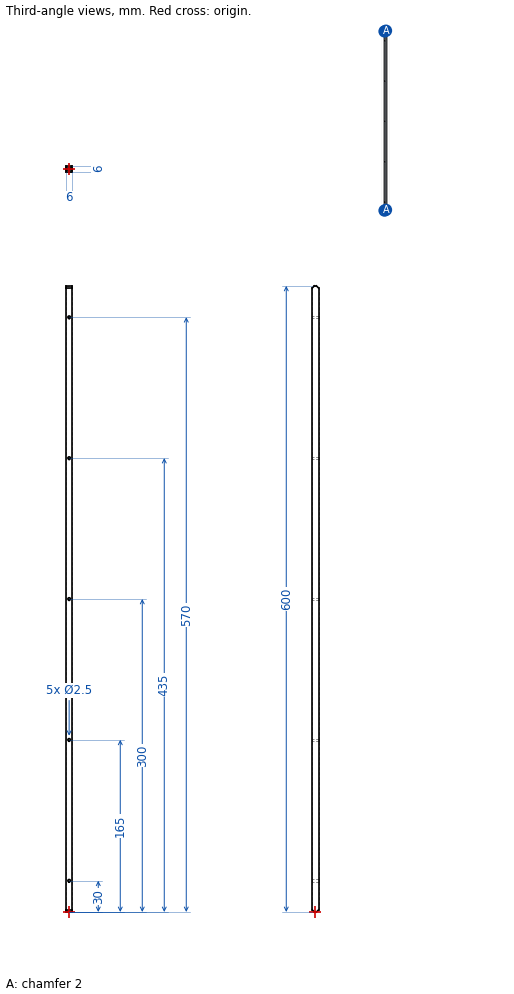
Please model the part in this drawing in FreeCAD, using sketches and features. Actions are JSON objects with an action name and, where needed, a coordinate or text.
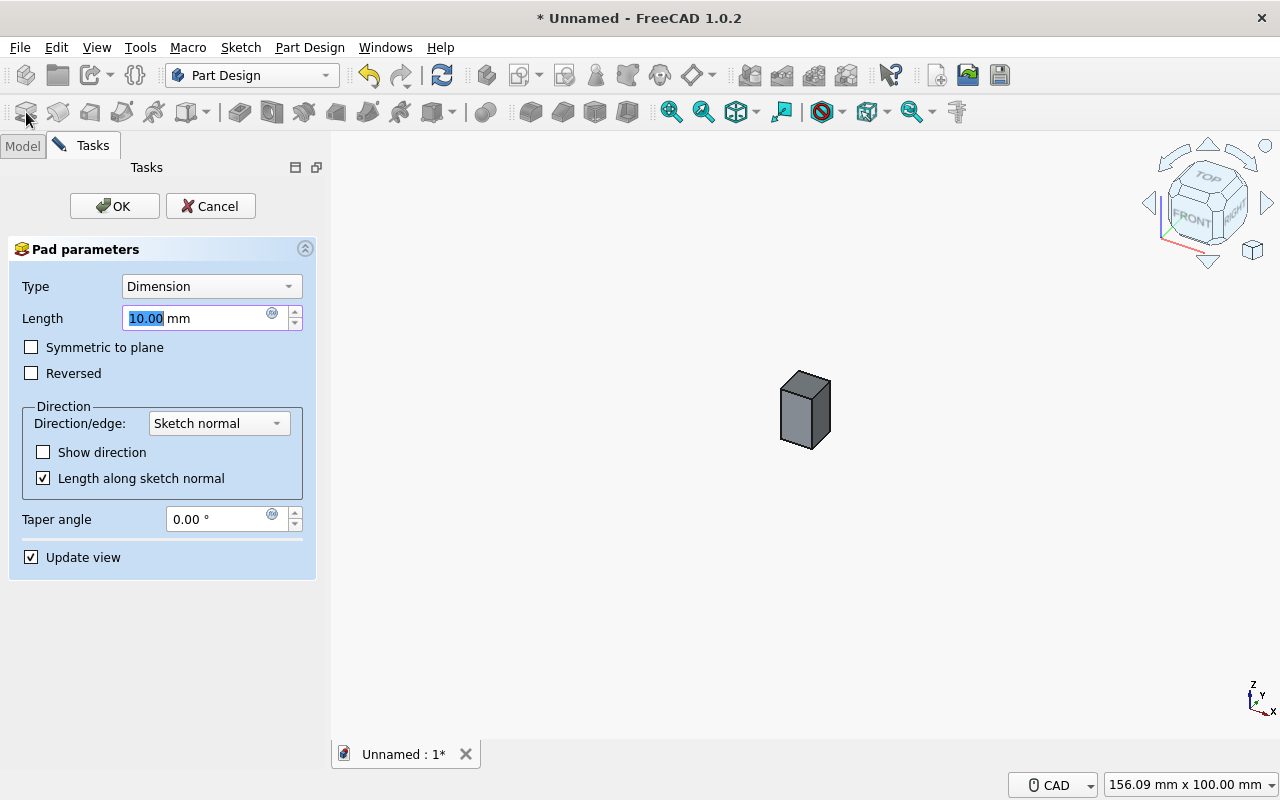
{"action": "type", "text": "600"}
{"action": "key", "text": "Tab"}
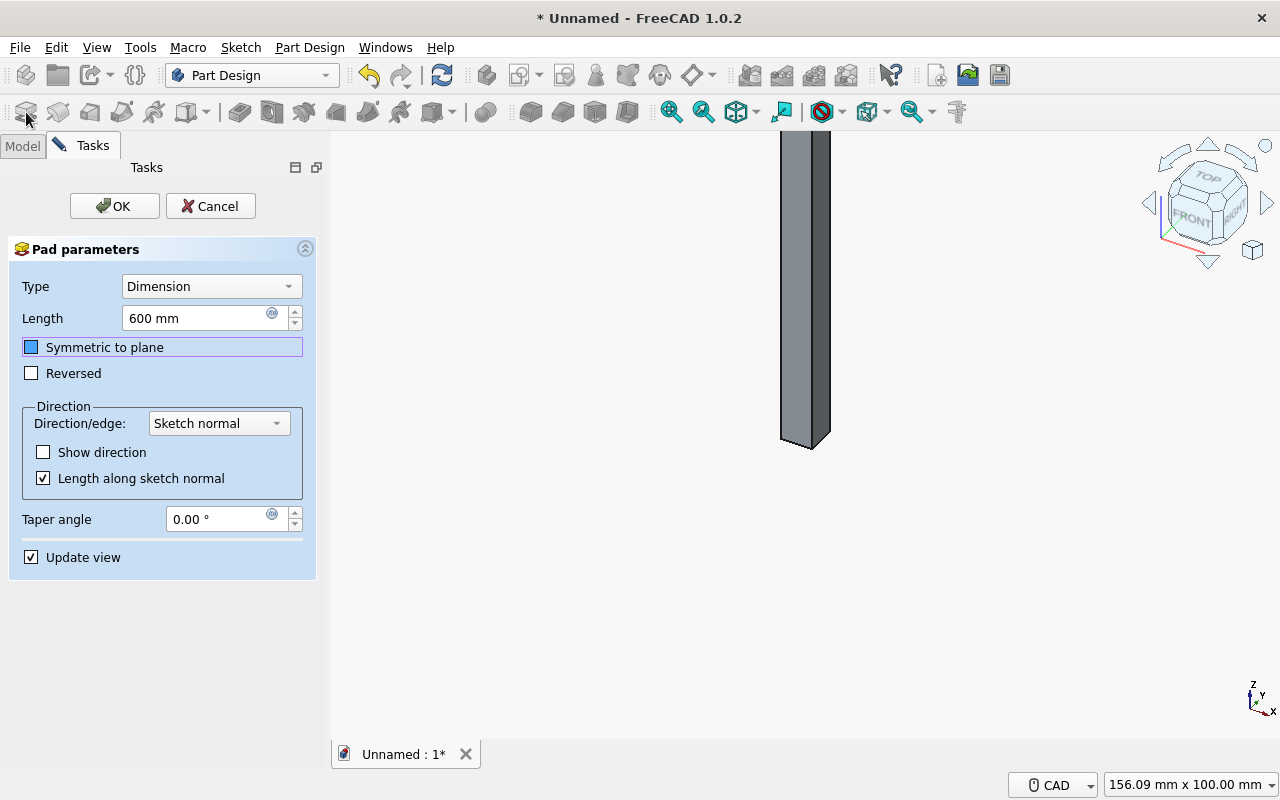
{"action": "left_click", "coordinate": [115, 206]}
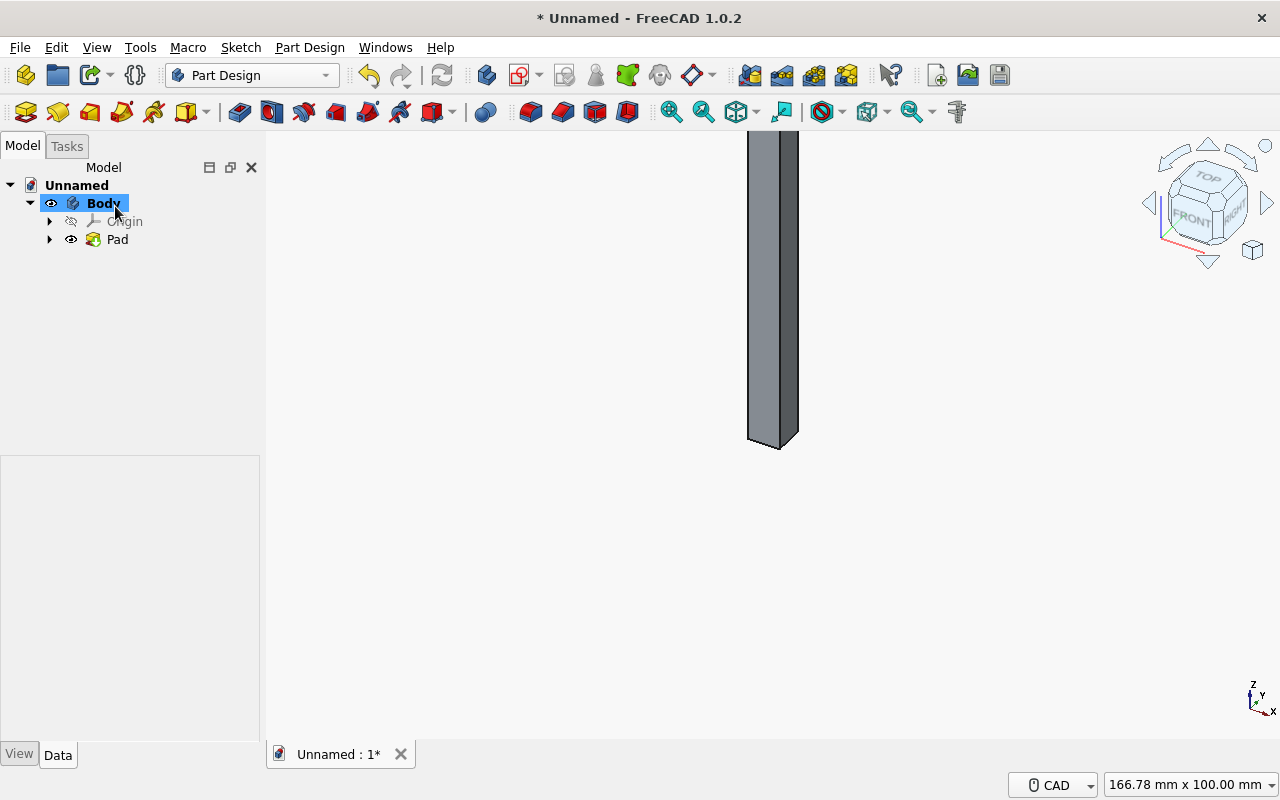
{"action": "left_click", "coordinate": [672, 112]}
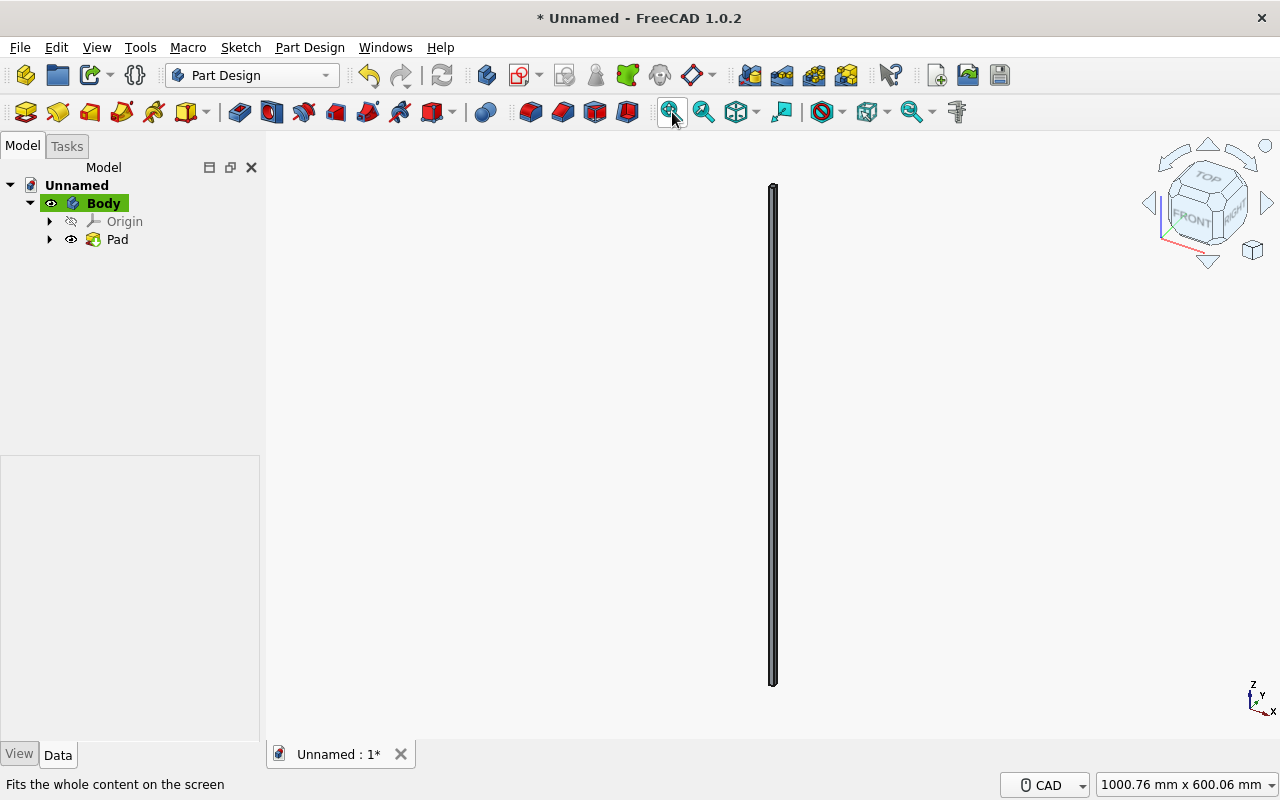
{"action": "key", "text": "4"}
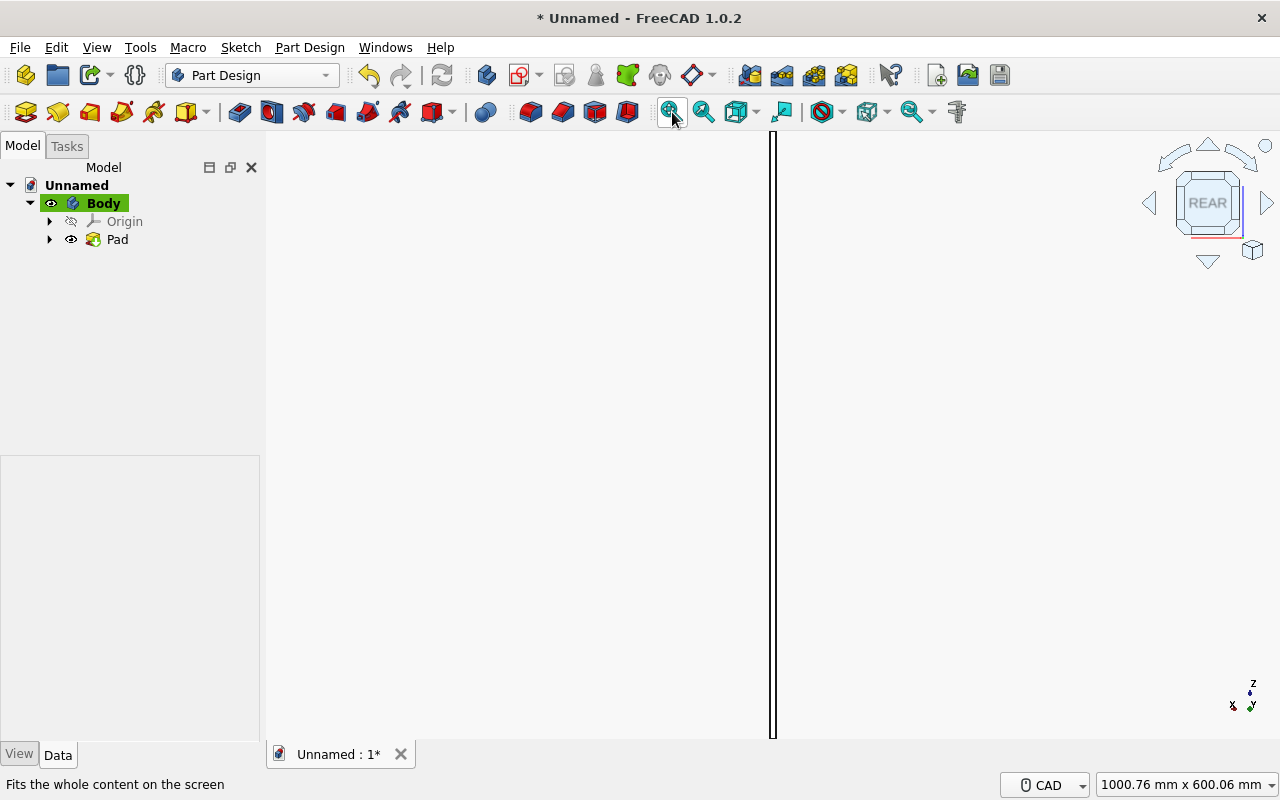
{"action": "left_click", "coordinate": [672, 112]}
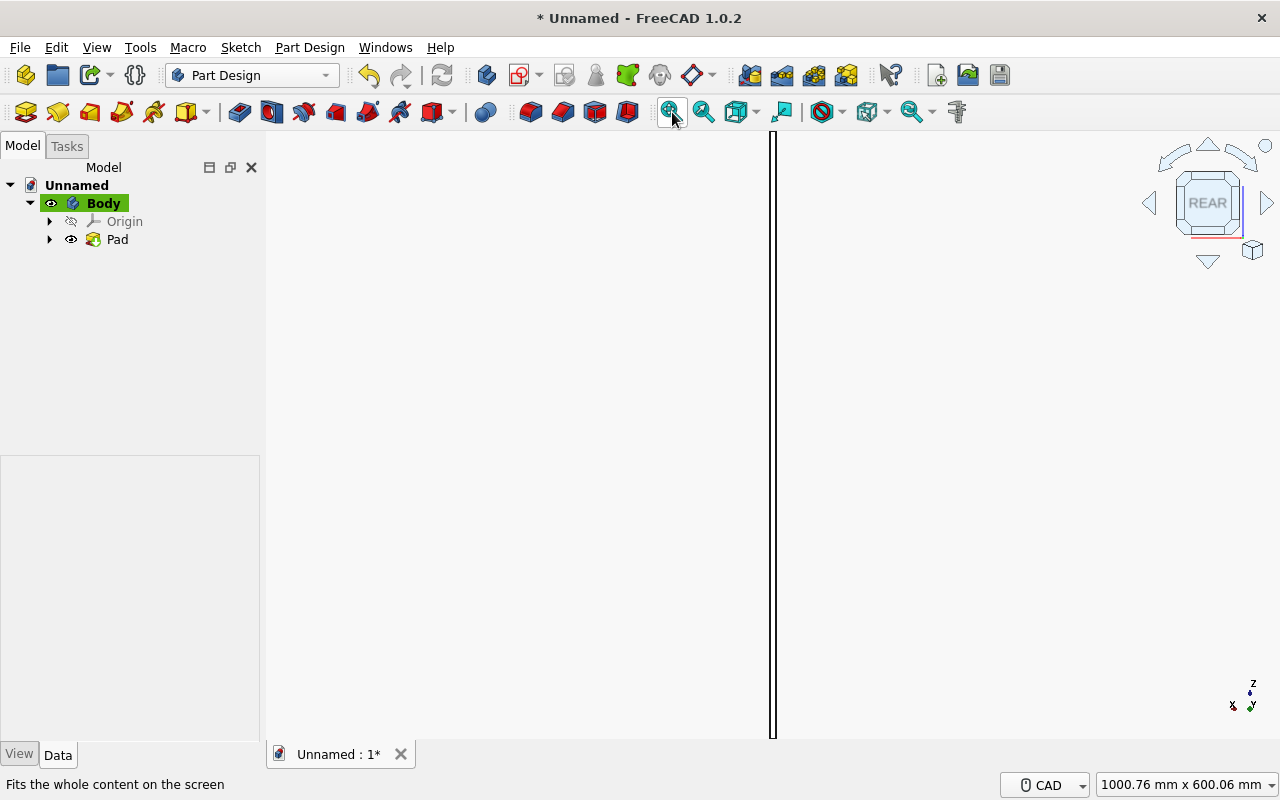
{"action": "scroll", "coordinate": [773, 173], "scroll_direction": "up", "scroll_amount": 7}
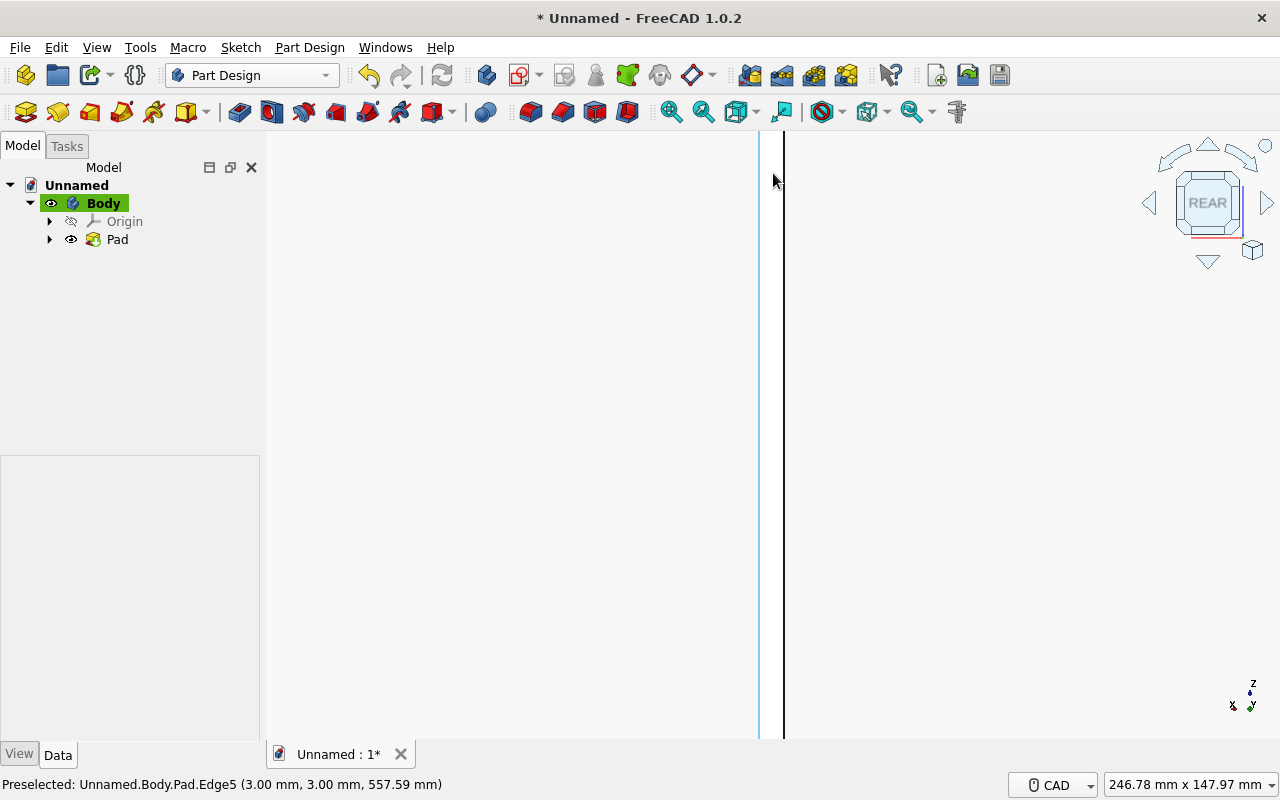
{"action": "left_click", "coordinate": [771, 178]}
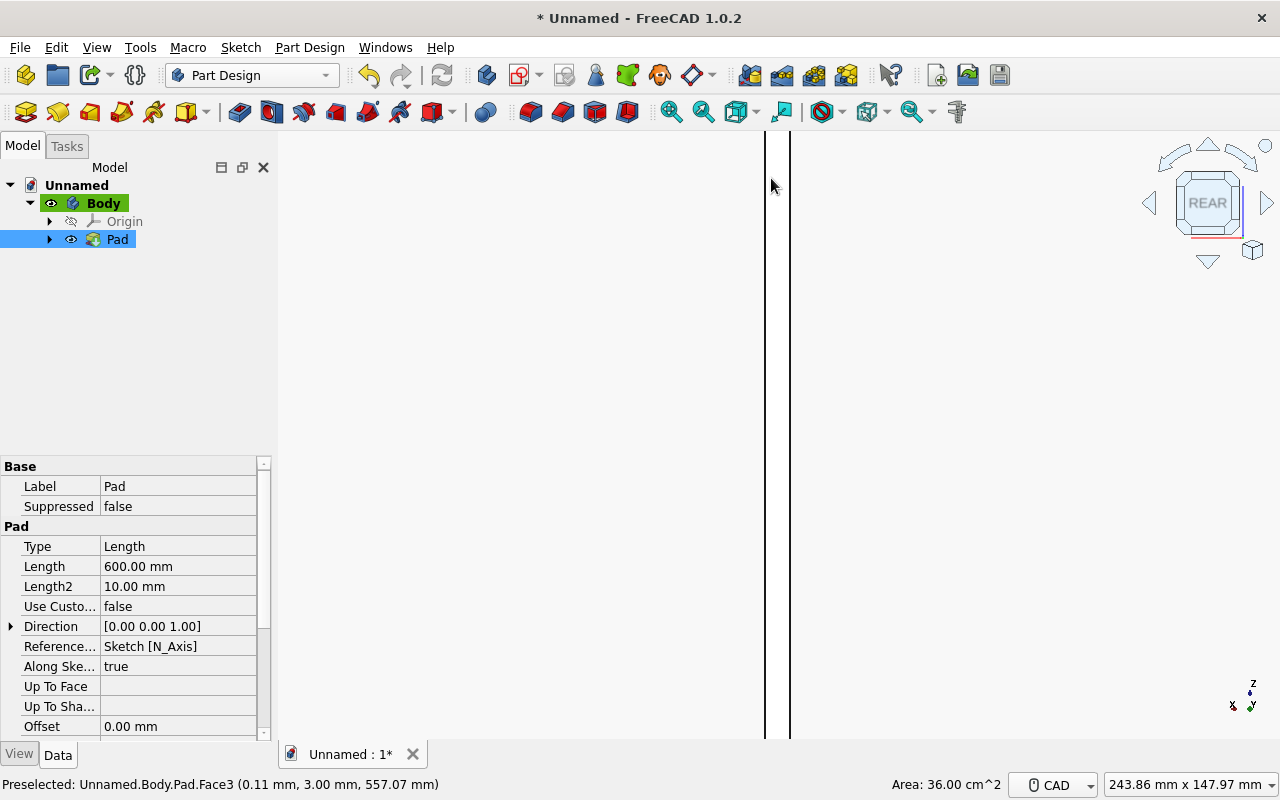
{"action": "left_click", "coordinate": [520, 76]}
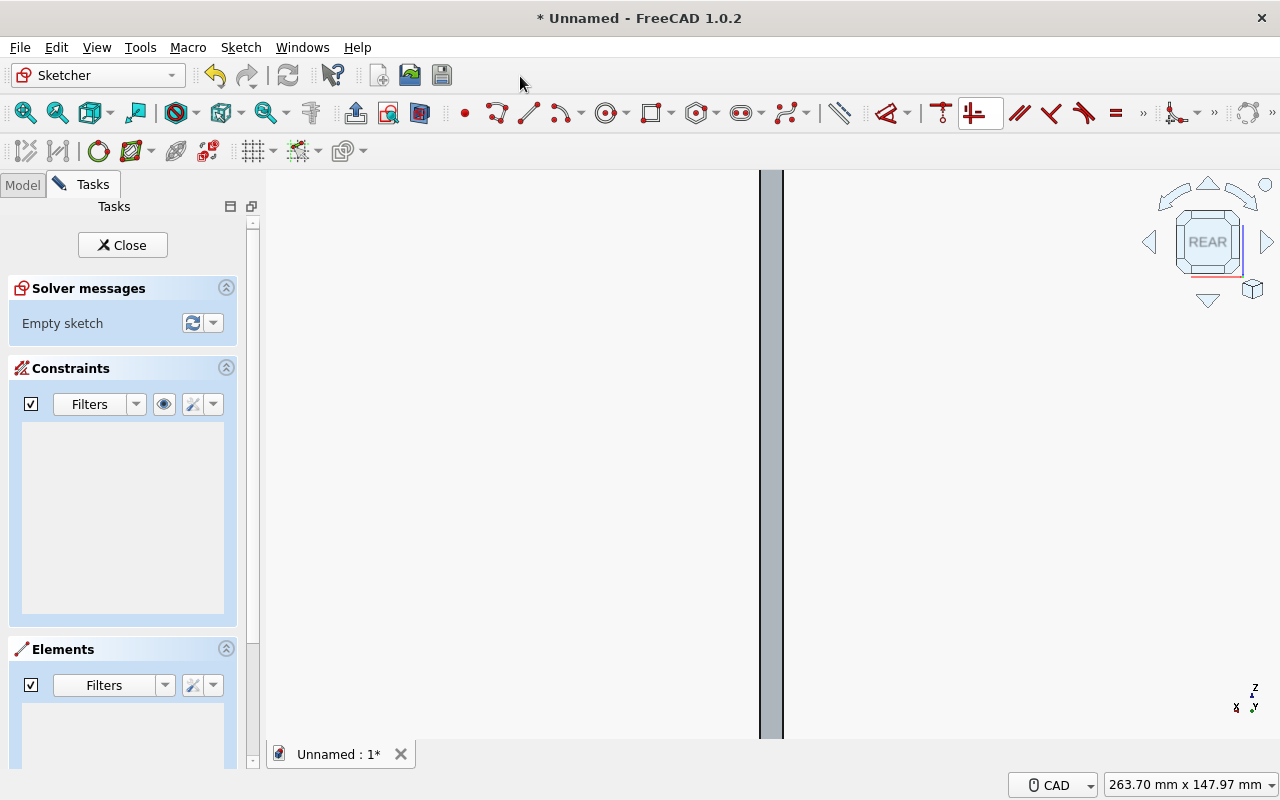
{"action": "scroll", "coordinate": [691, 295], "scroll_direction": "down", "scroll_amount": 9}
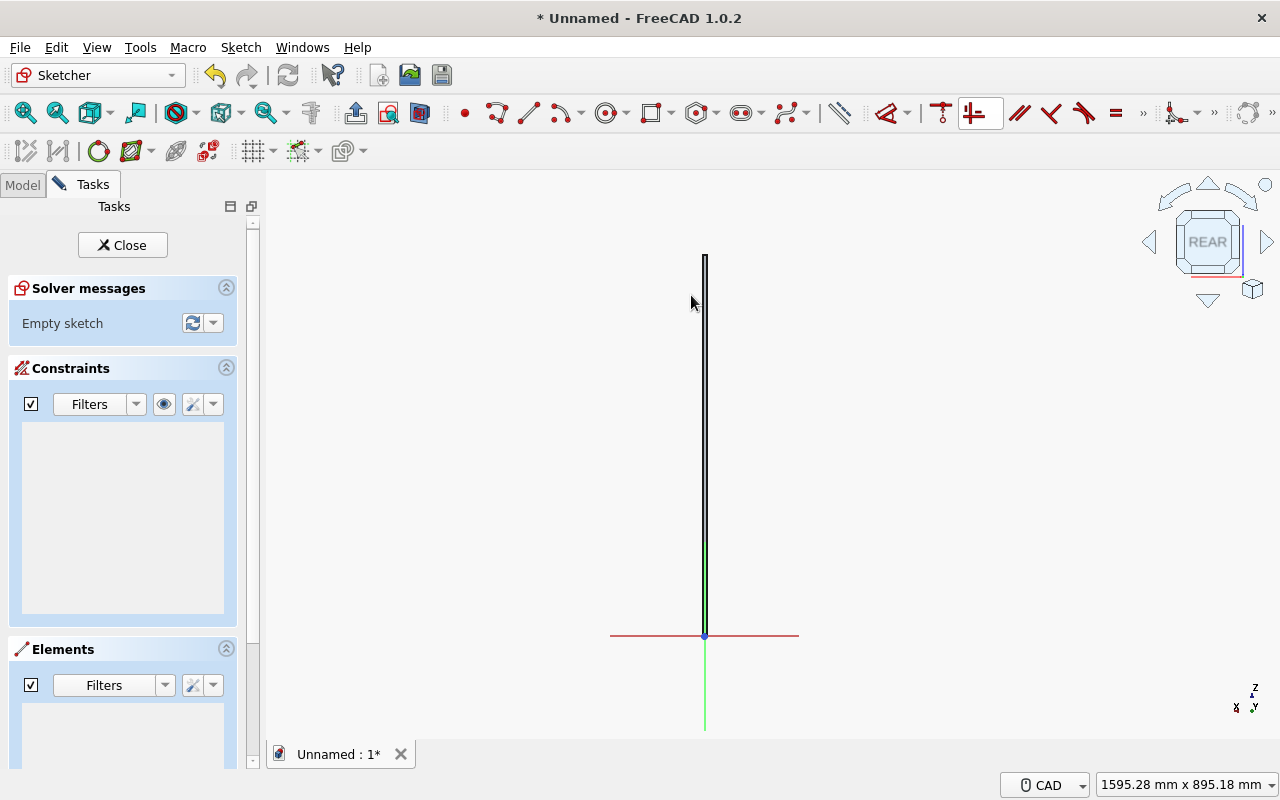
{"action": "left_click", "coordinate": [606, 114]}